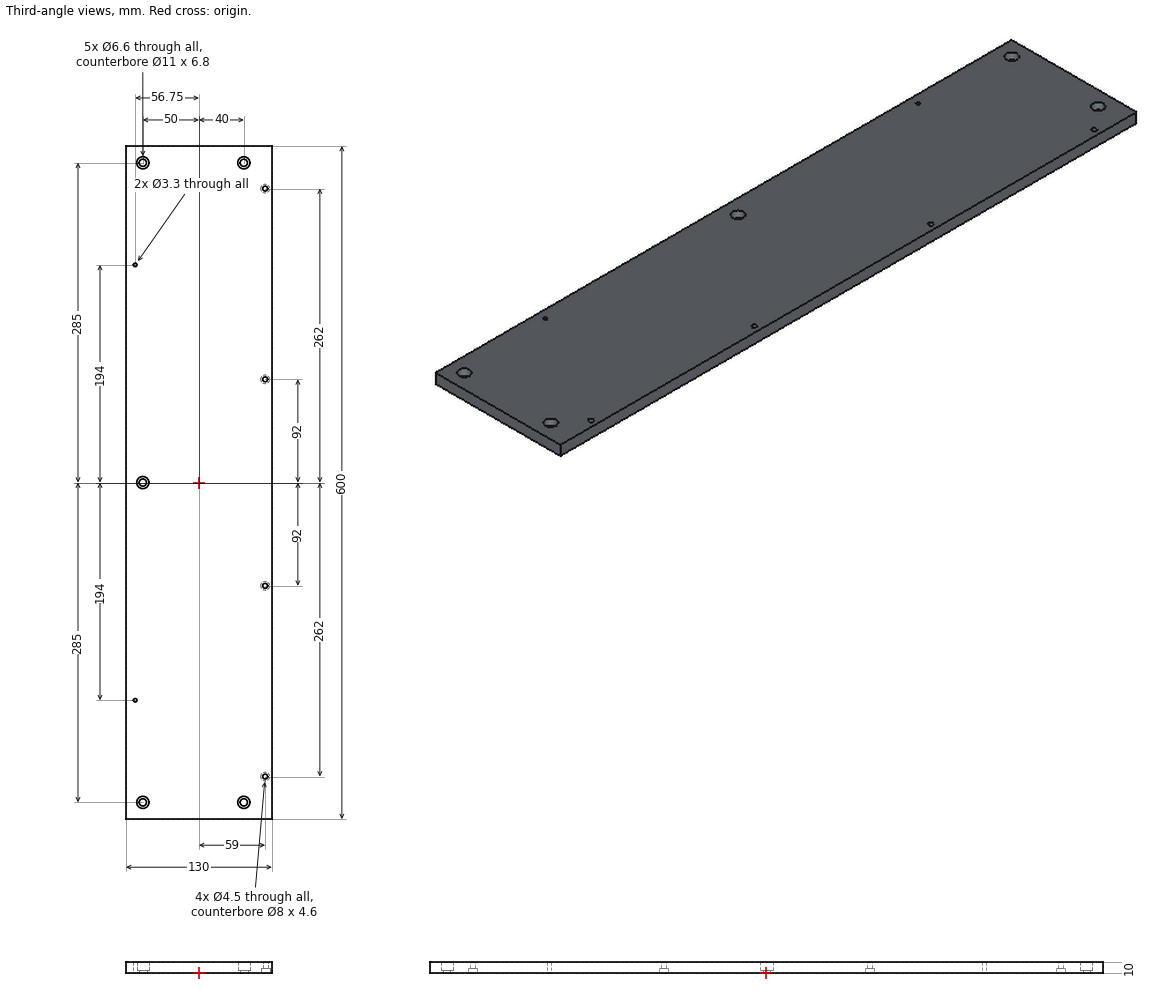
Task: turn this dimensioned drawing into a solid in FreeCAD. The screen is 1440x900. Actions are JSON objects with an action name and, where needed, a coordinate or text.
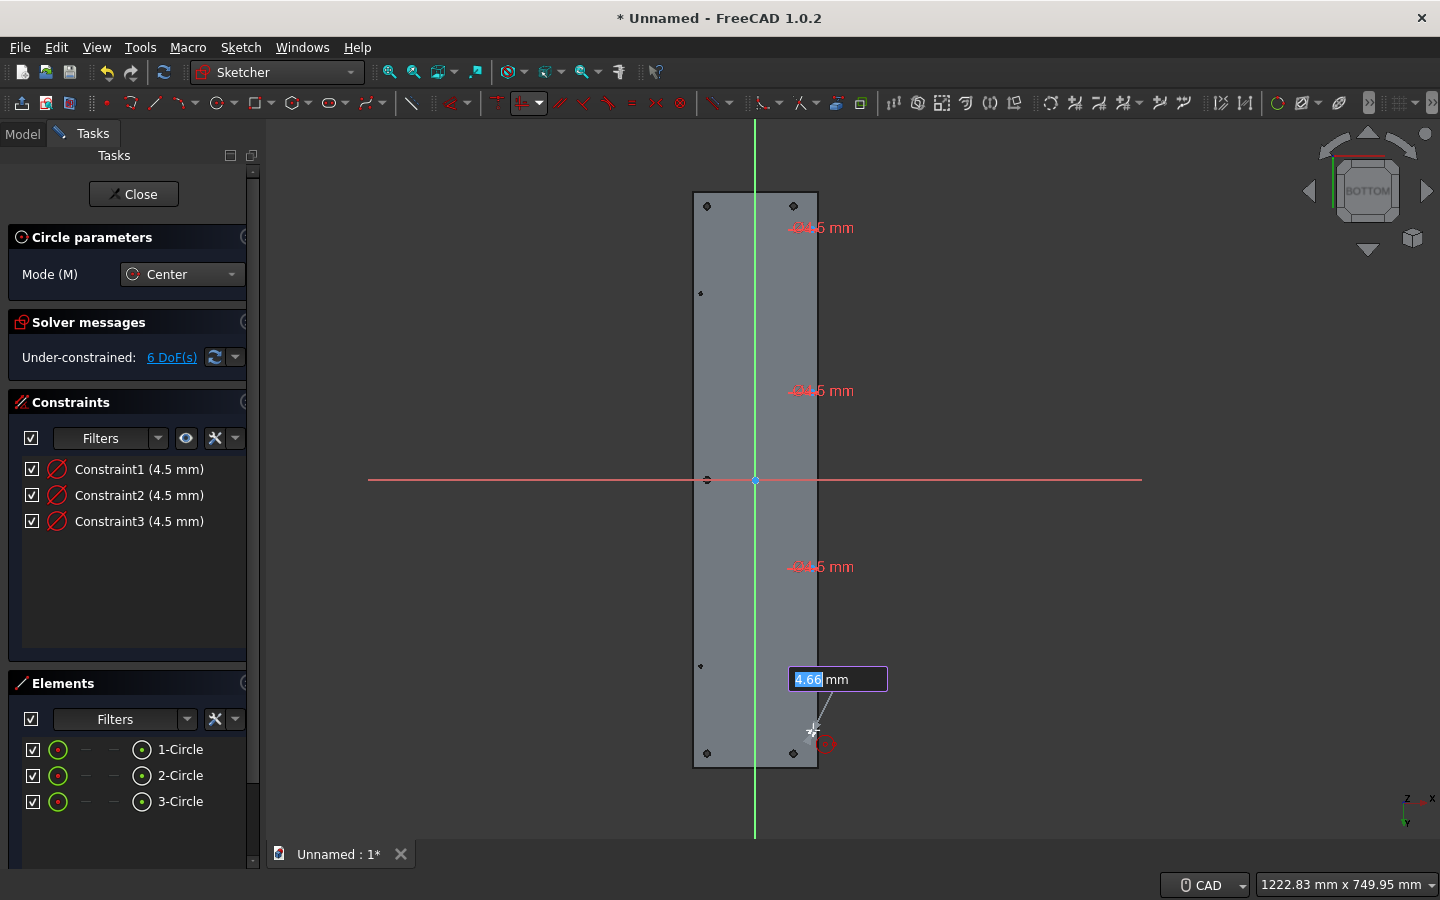
{"action": "type", "text": "4.5"}
{"action": "key", "text": "Return"}
{"action": "key", "text": "Escape"}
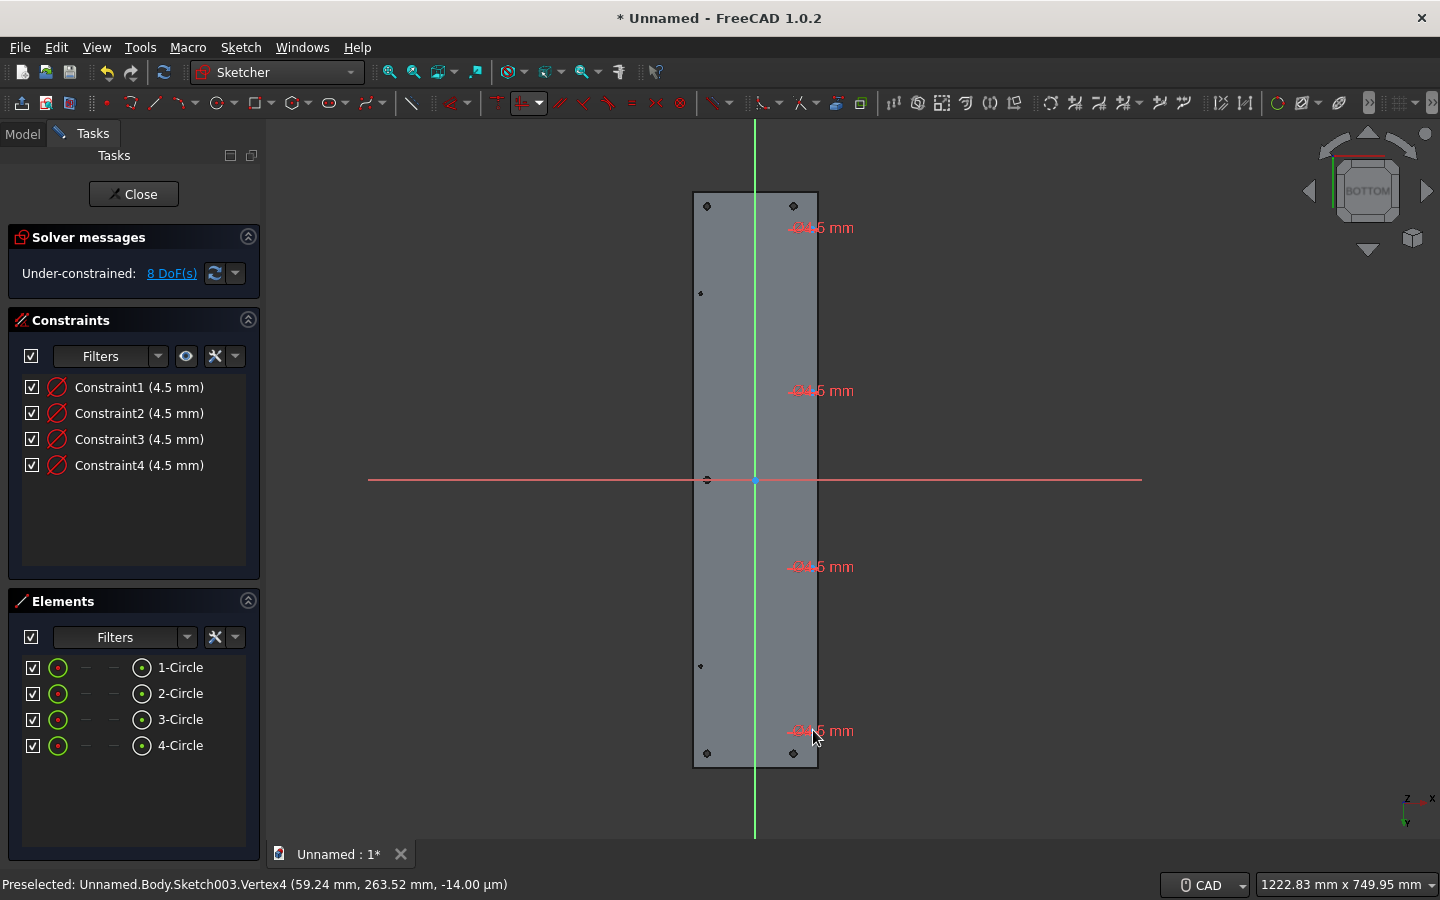
{"action": "left_click", "coordinate": [812, 230]}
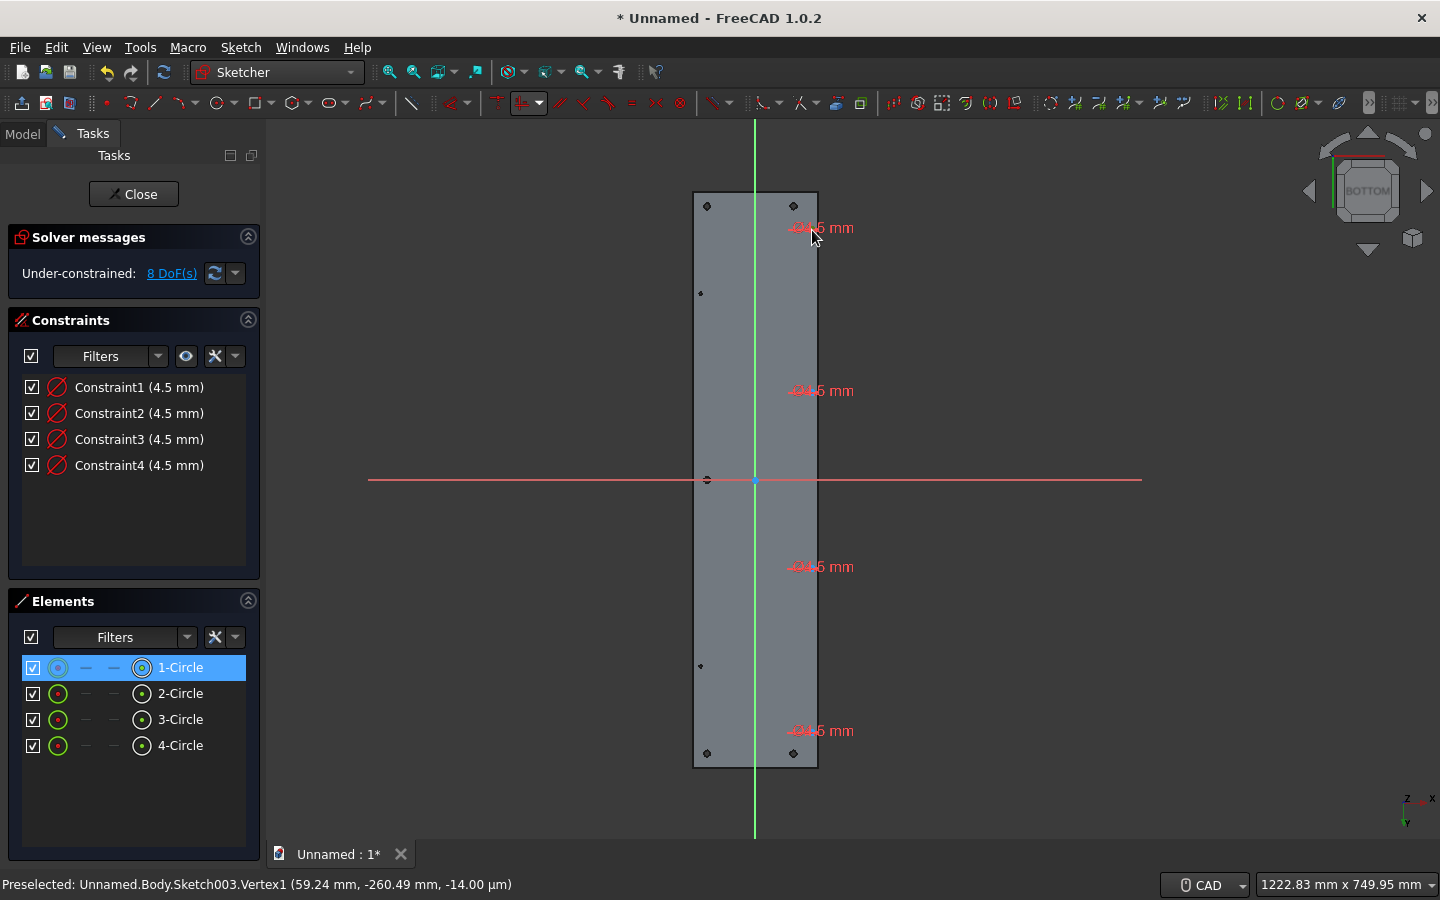
{"action": "left_click", "coordinate": [812, 393]}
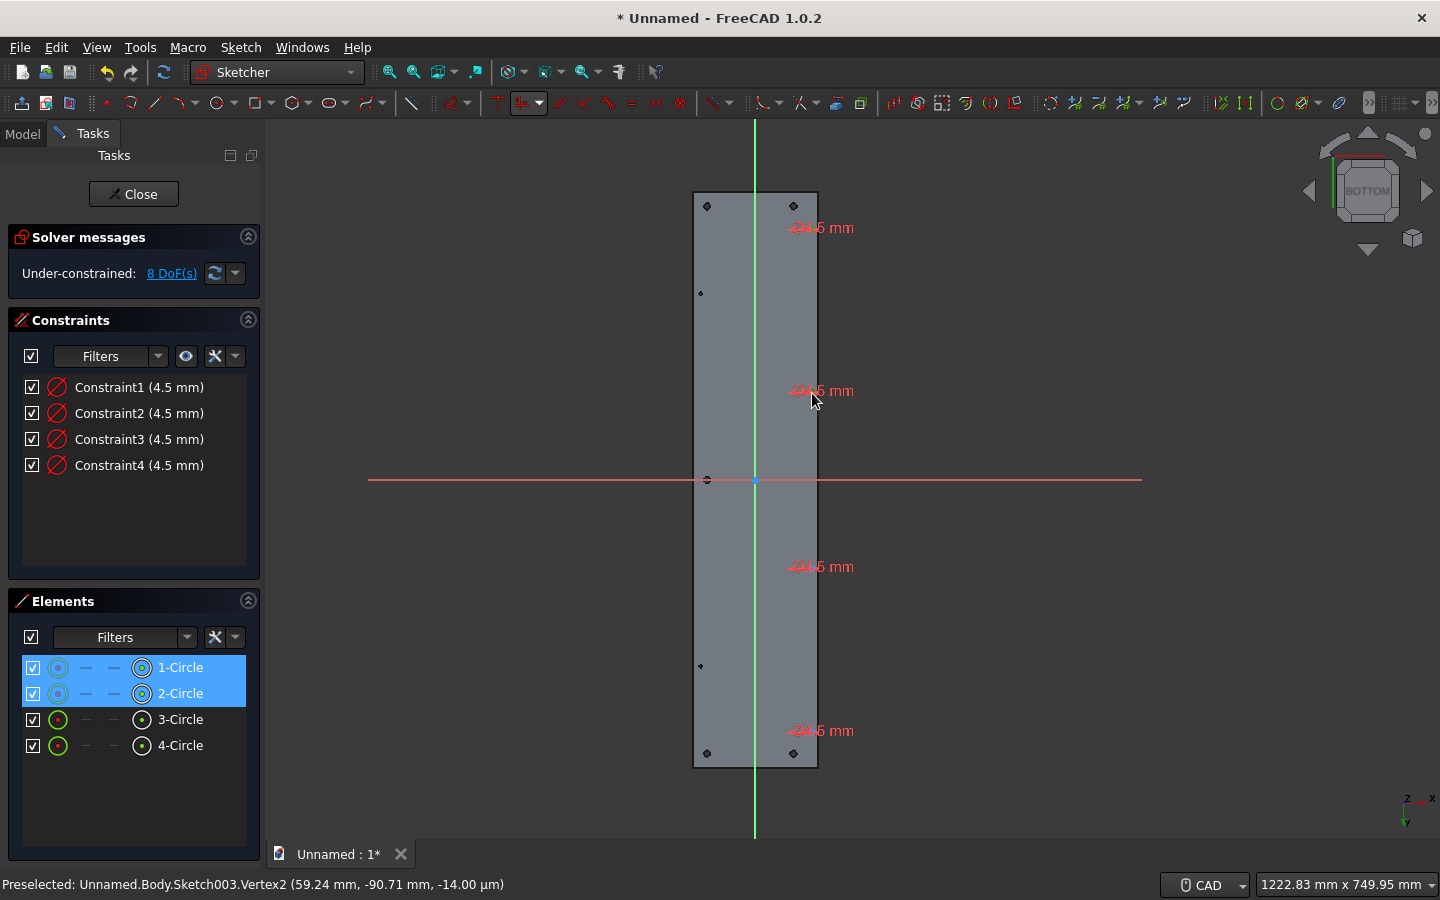
{"action": "key", "text": "v"}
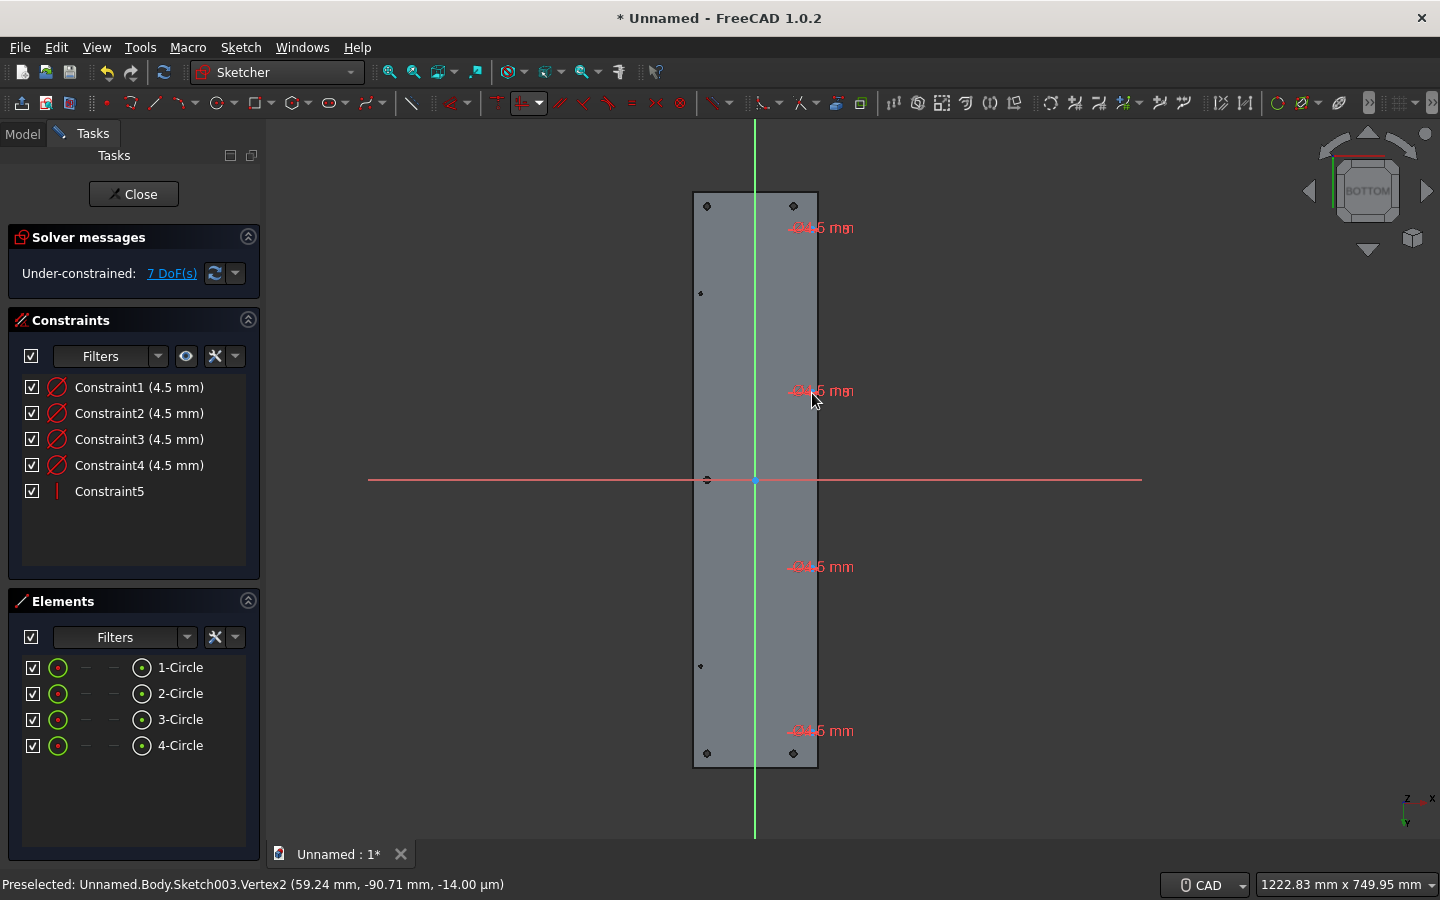
{"action": "left_click", "coordinate": [812, 393]}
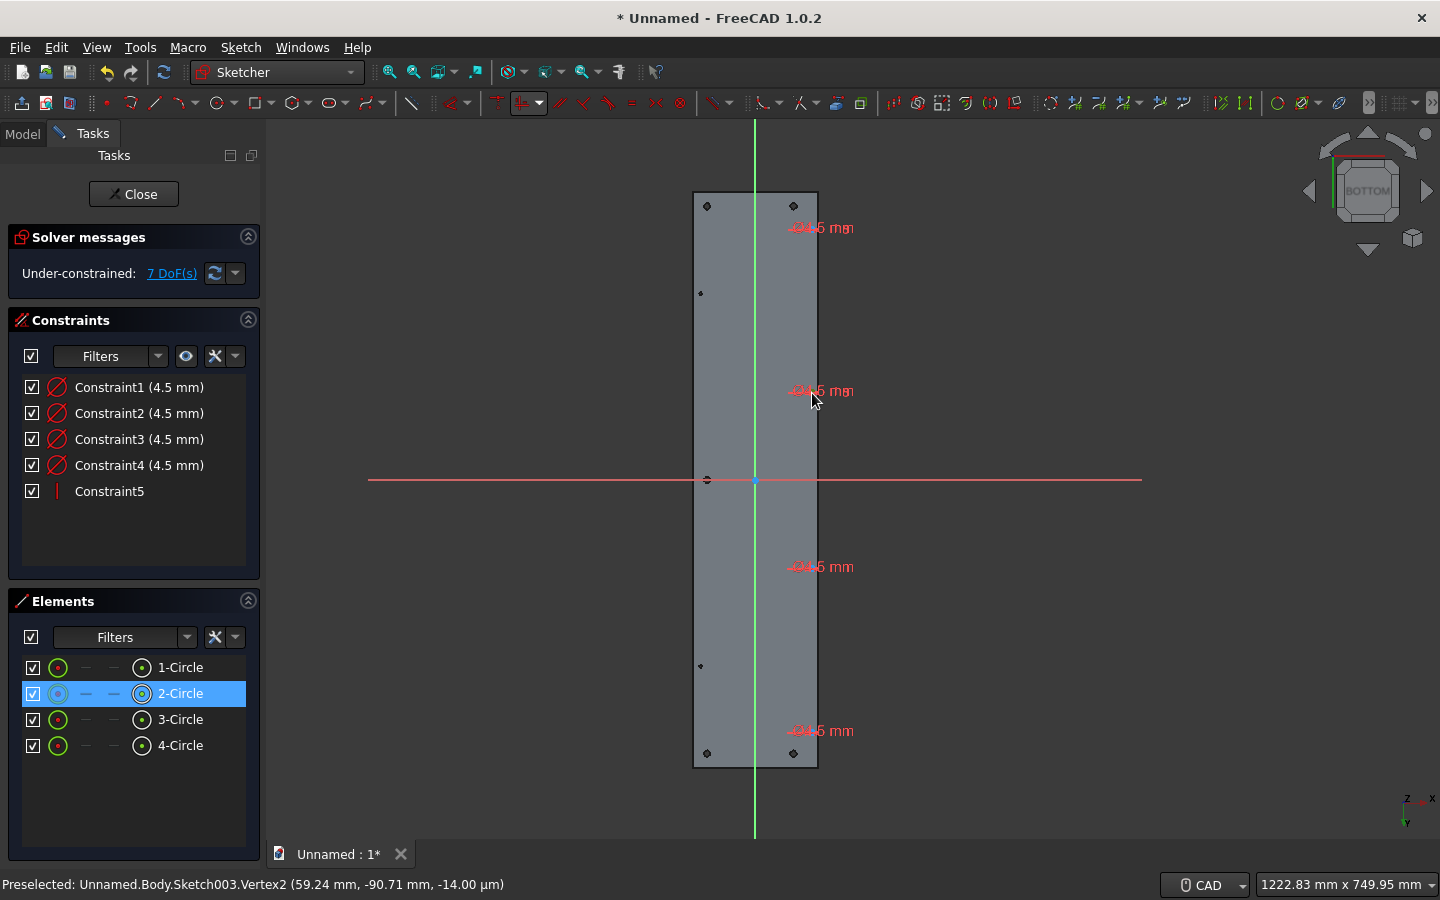
{"action": "left_click", "coordinate": [812, 569]}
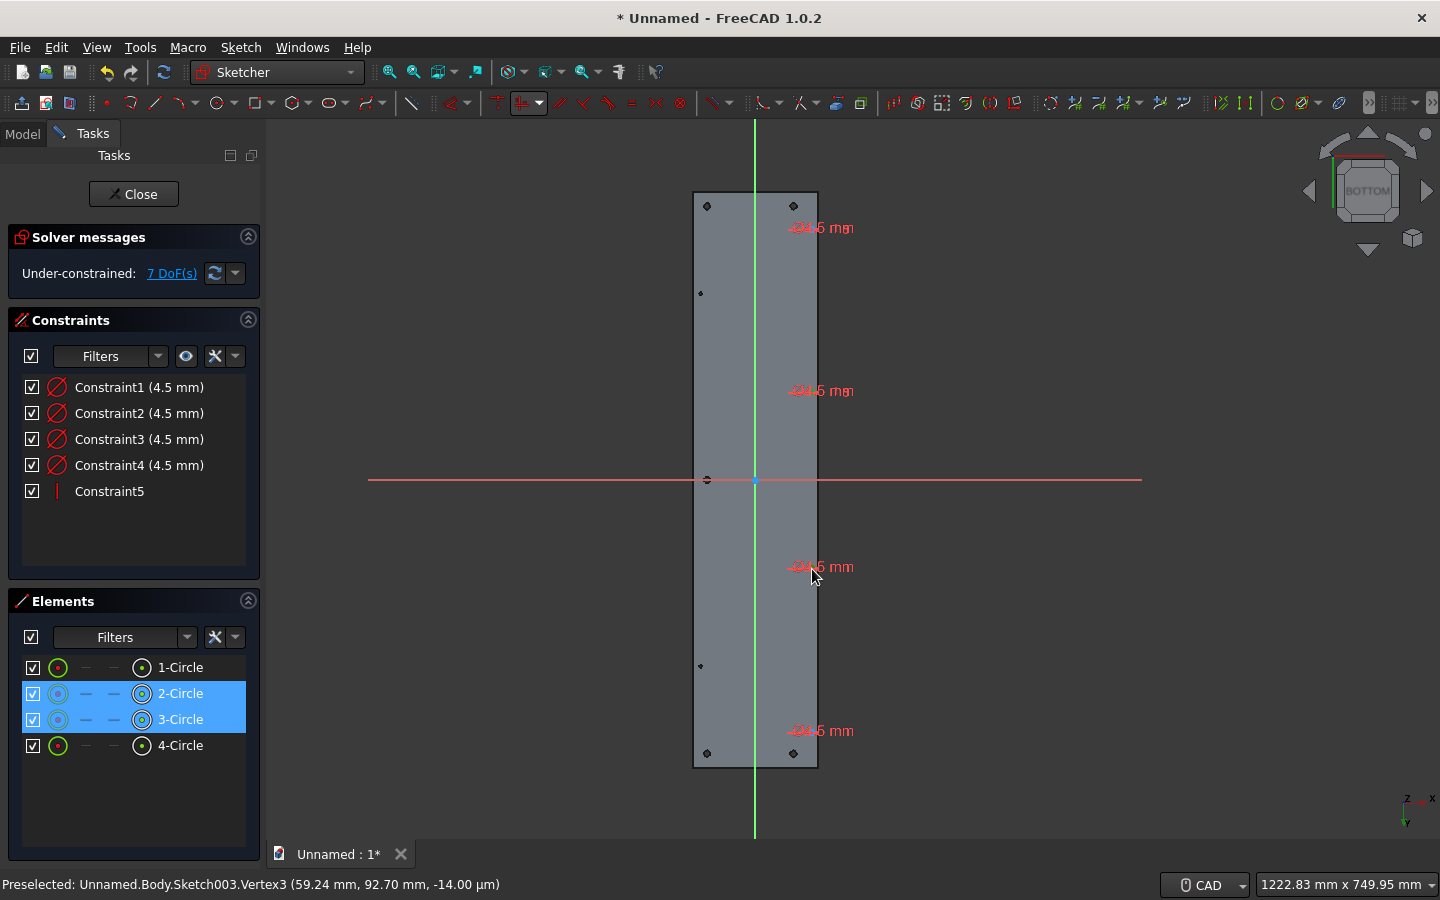
{"action": "left_click", "coordinate": [542, 104]}